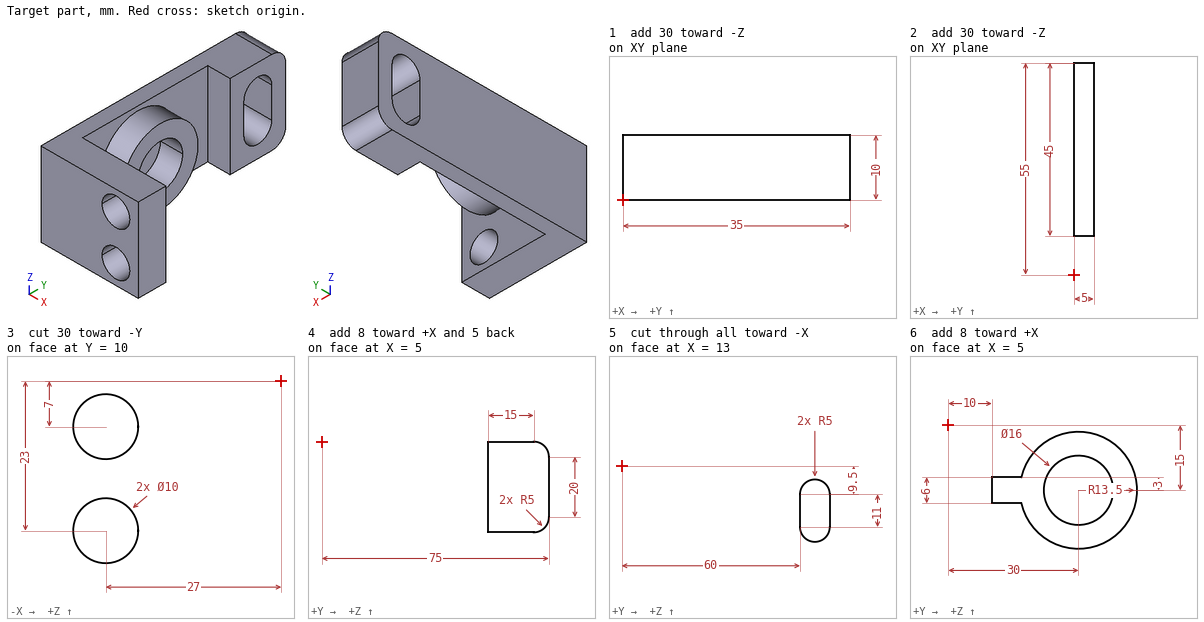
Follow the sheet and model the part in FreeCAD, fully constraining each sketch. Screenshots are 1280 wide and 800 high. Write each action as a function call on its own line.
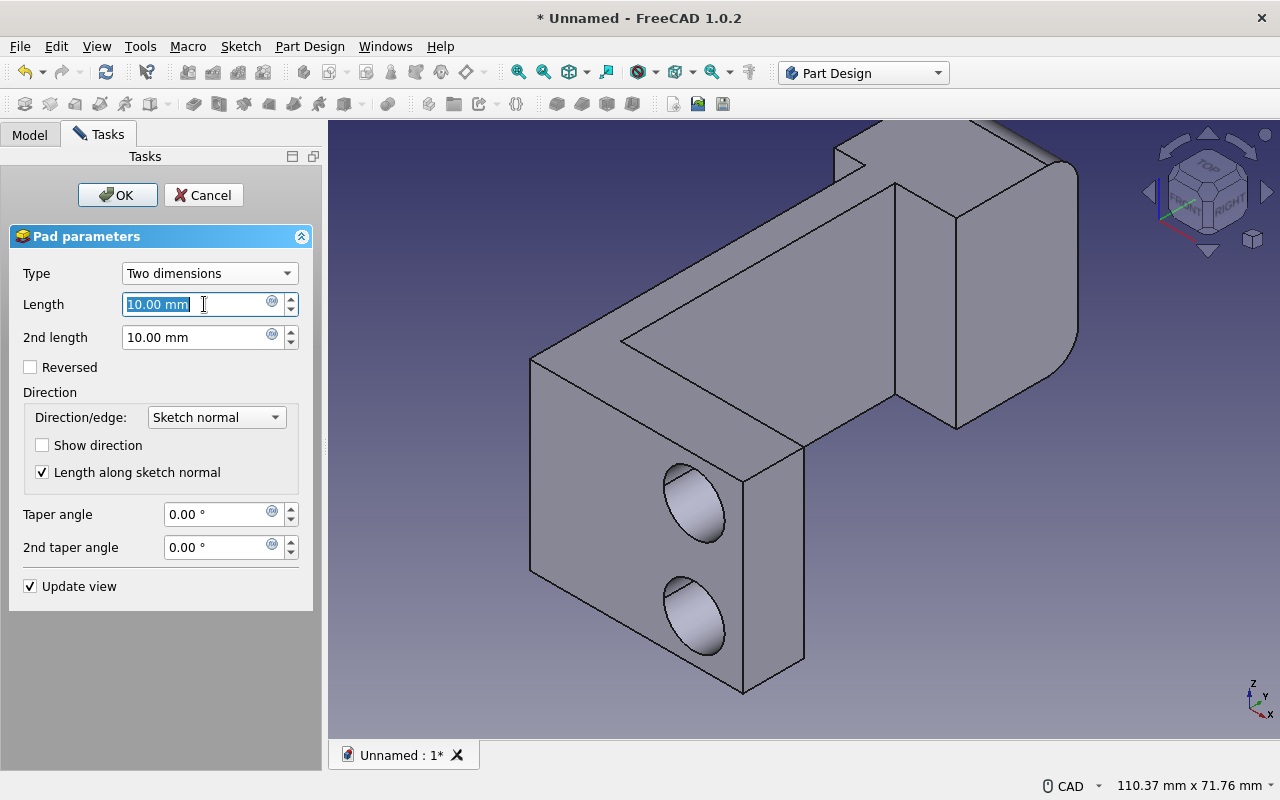
text(8)
key(Tab)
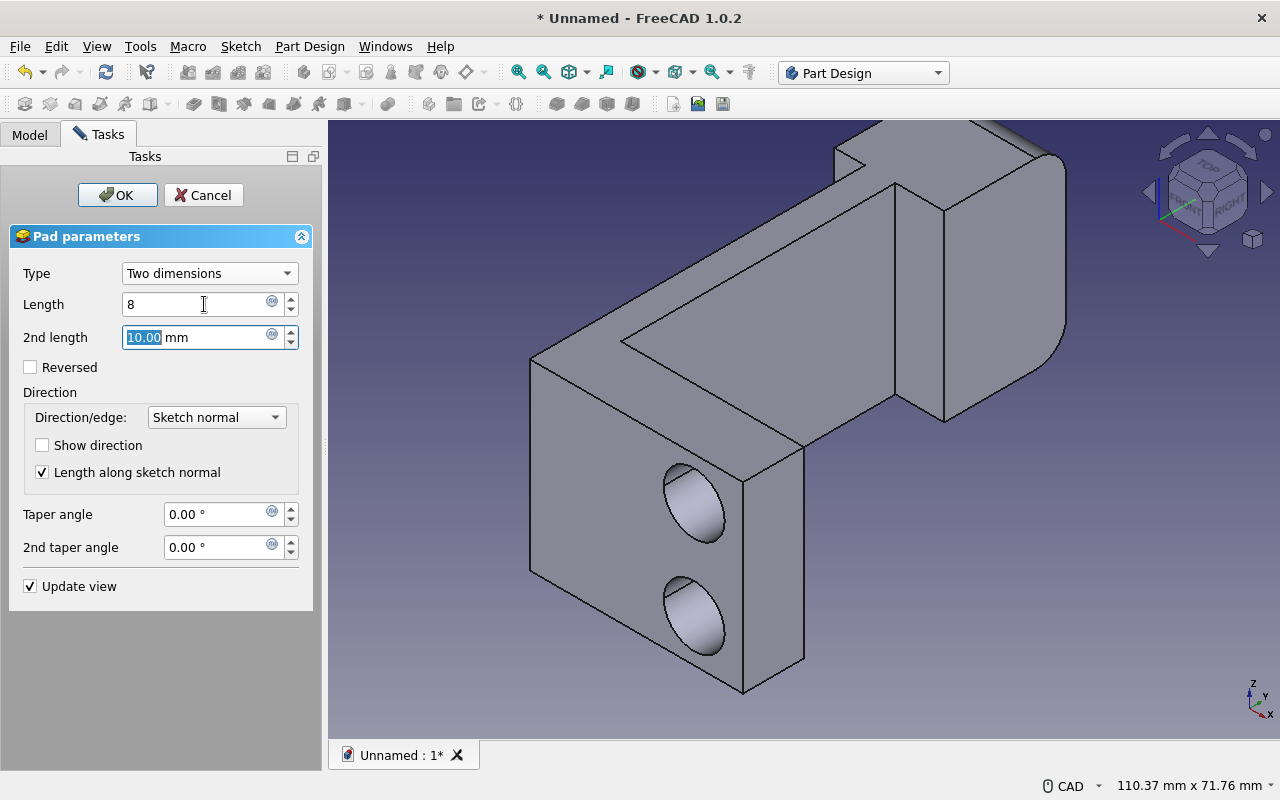
text(5)
key(Tab)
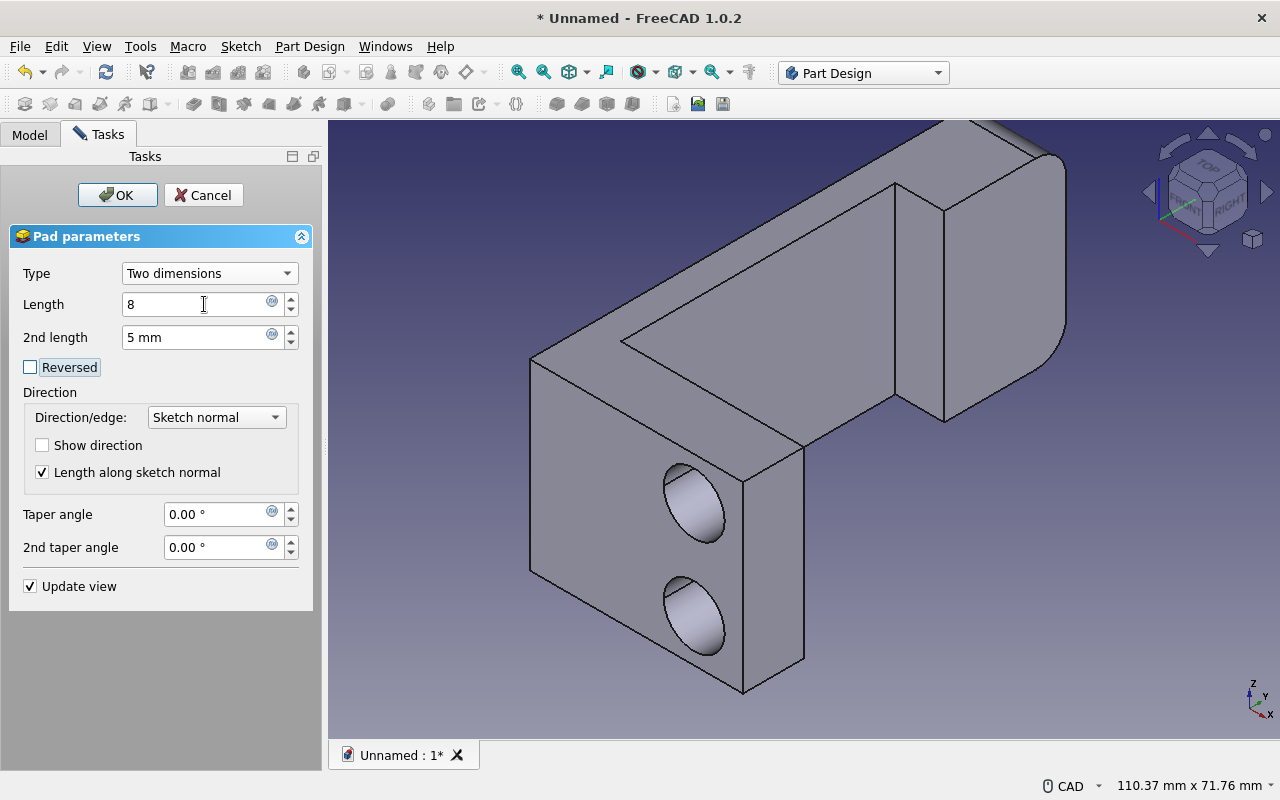
click(118, 195)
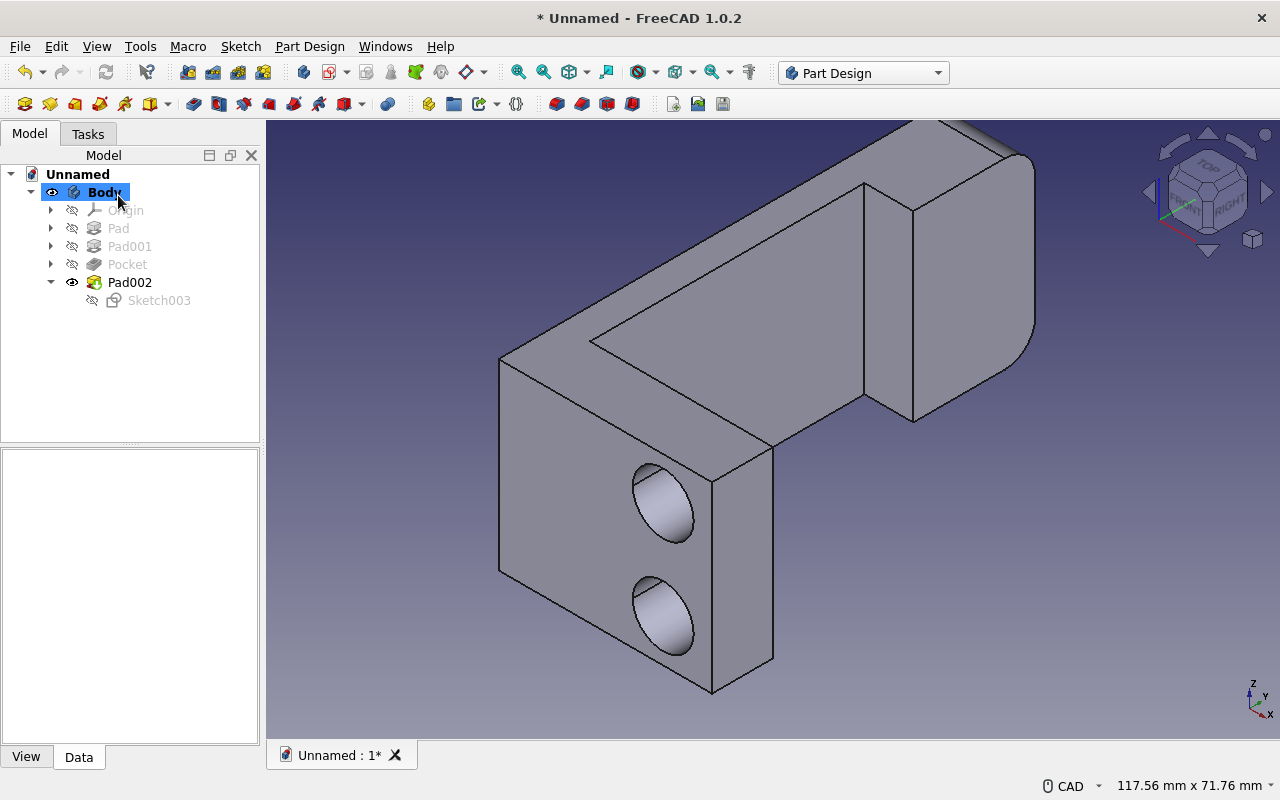
key(v)
key(f)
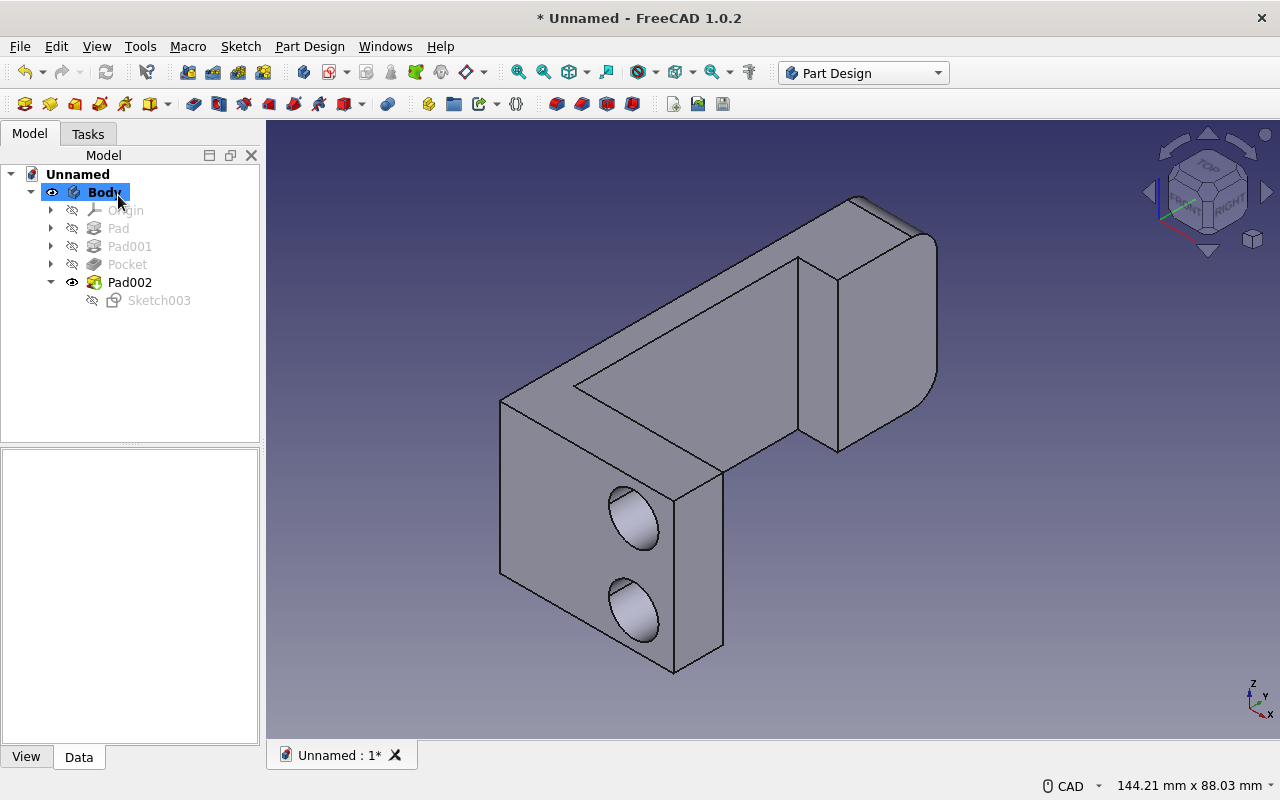
click(887, 312)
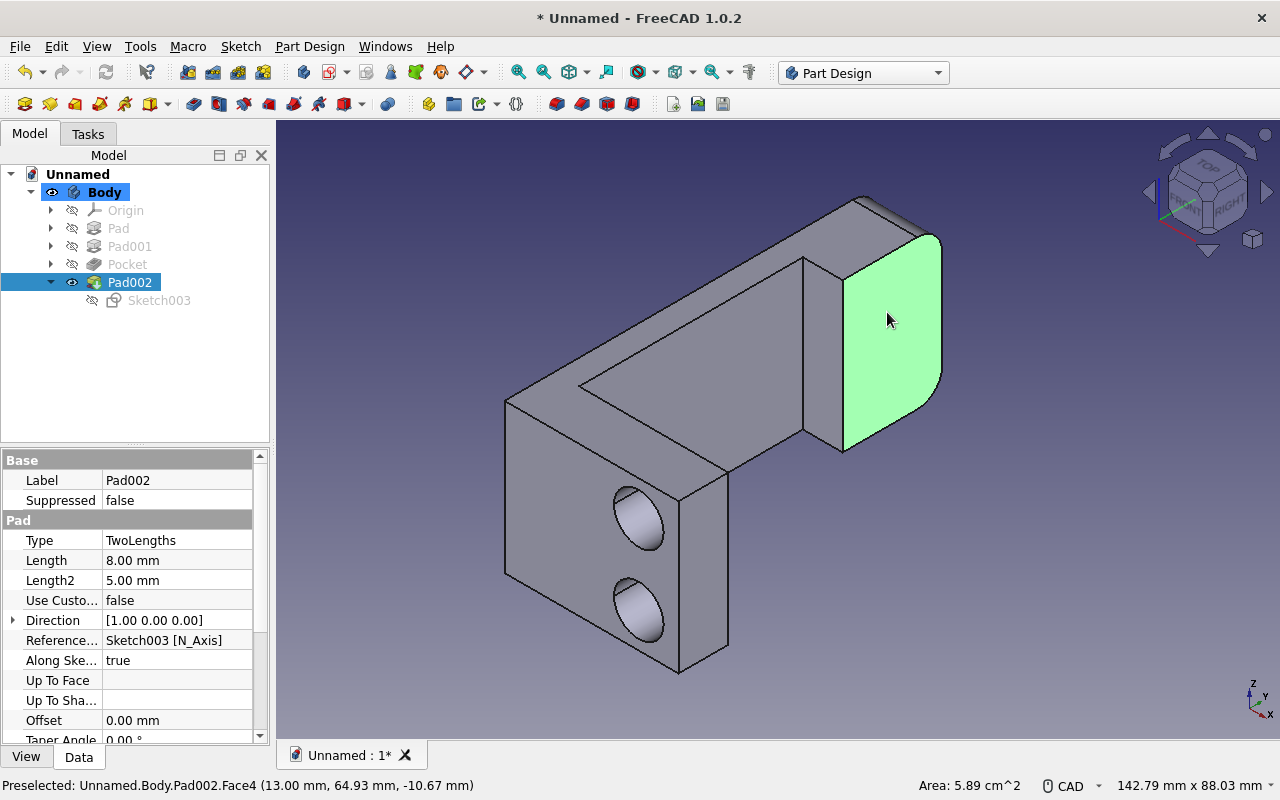
click(328, 72)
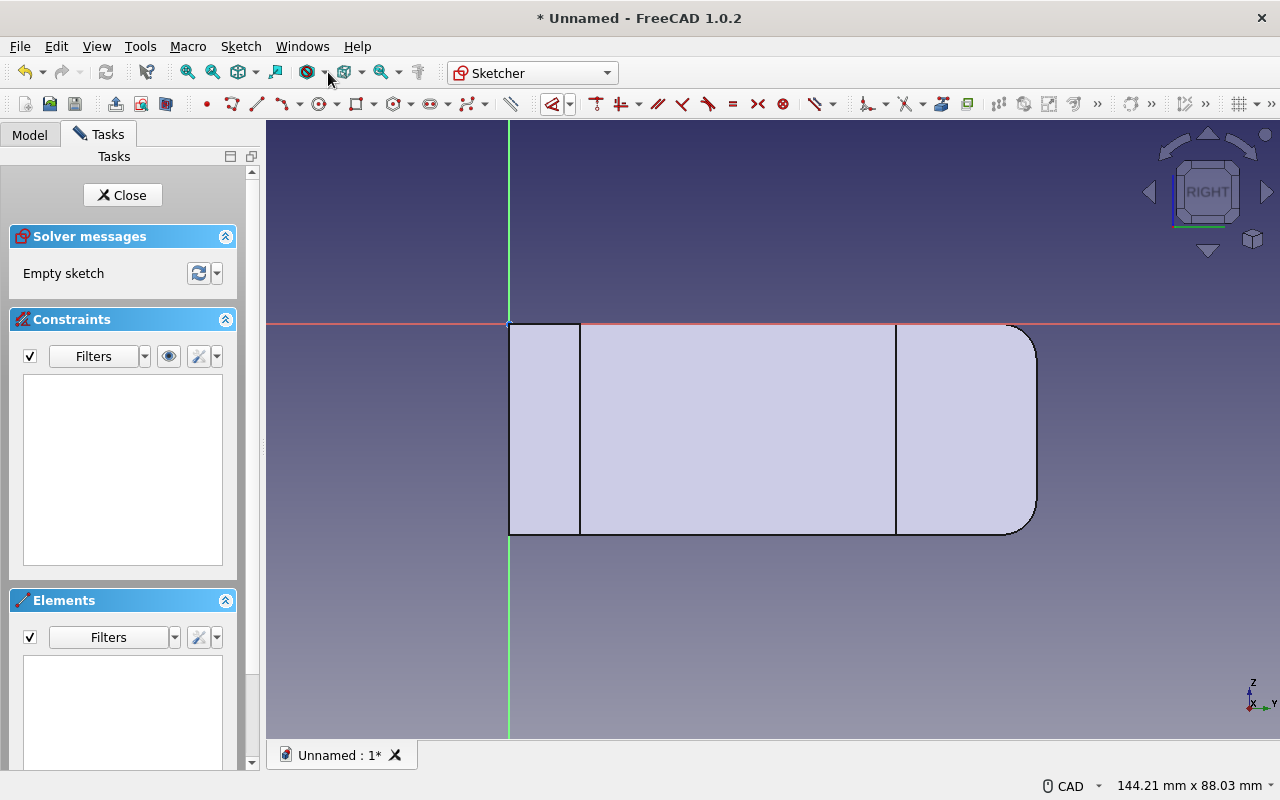
scroll(1115, 429, up, 5)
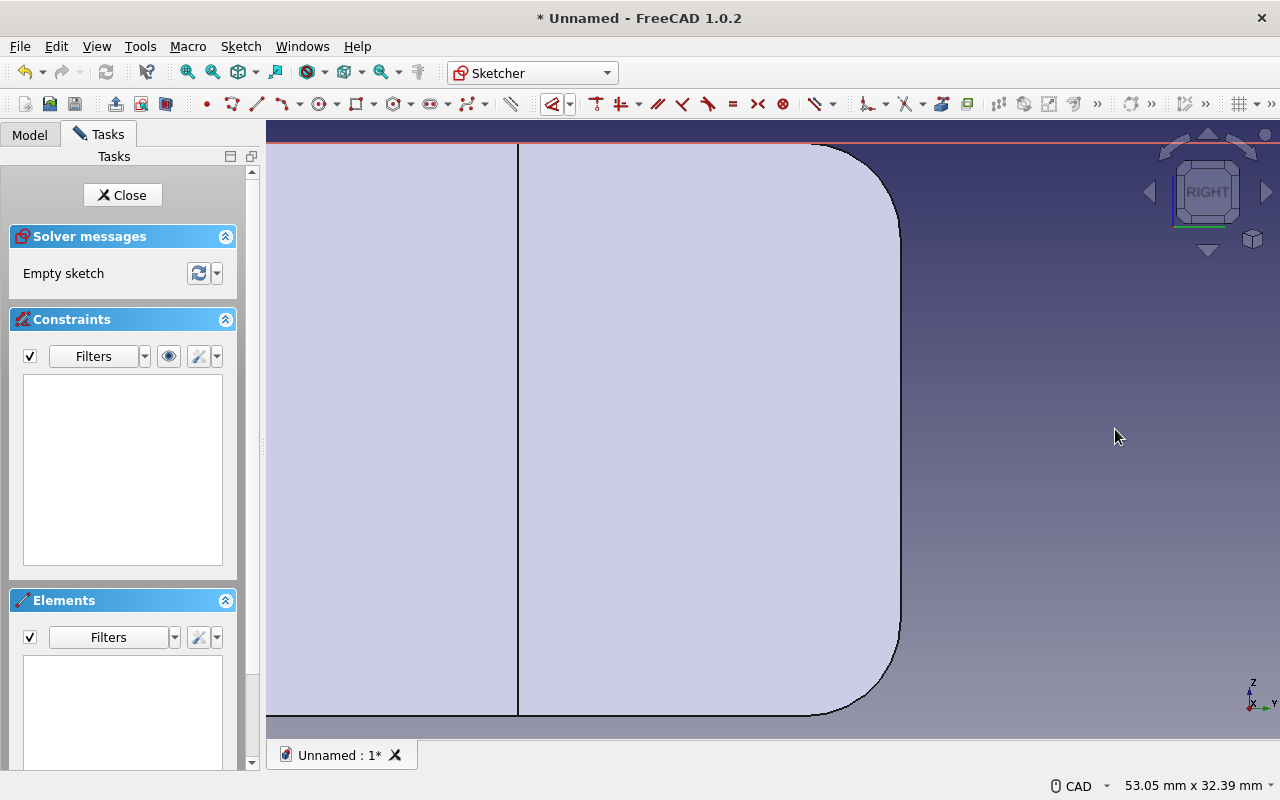
click(430, 104)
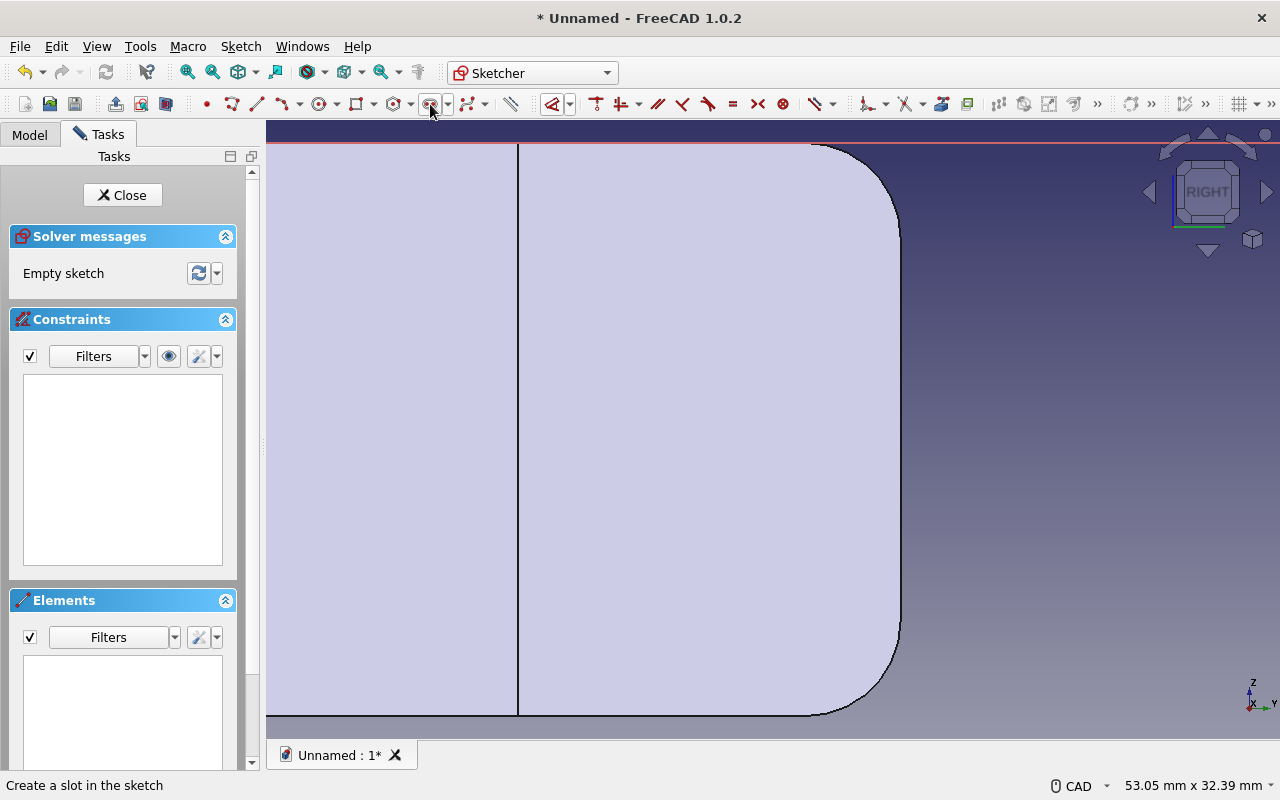
click(710, 535)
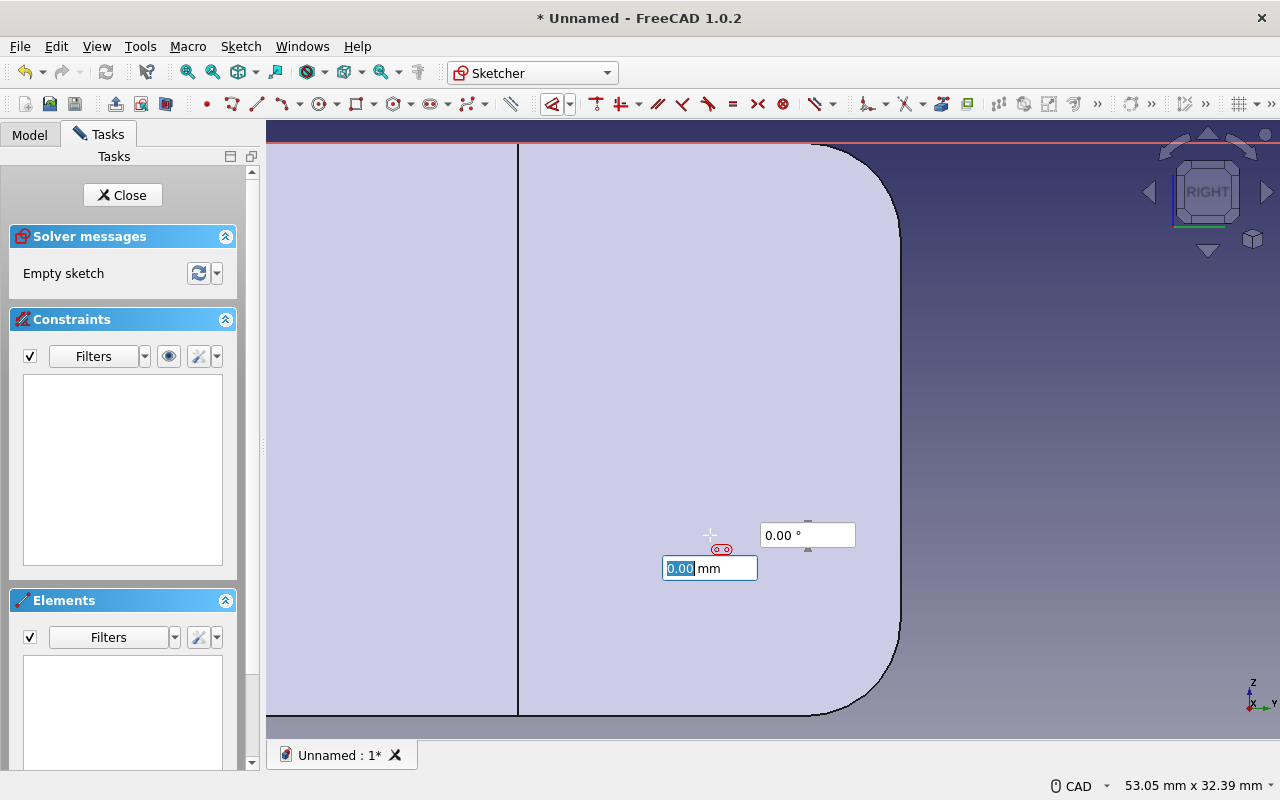
click(710, 324)